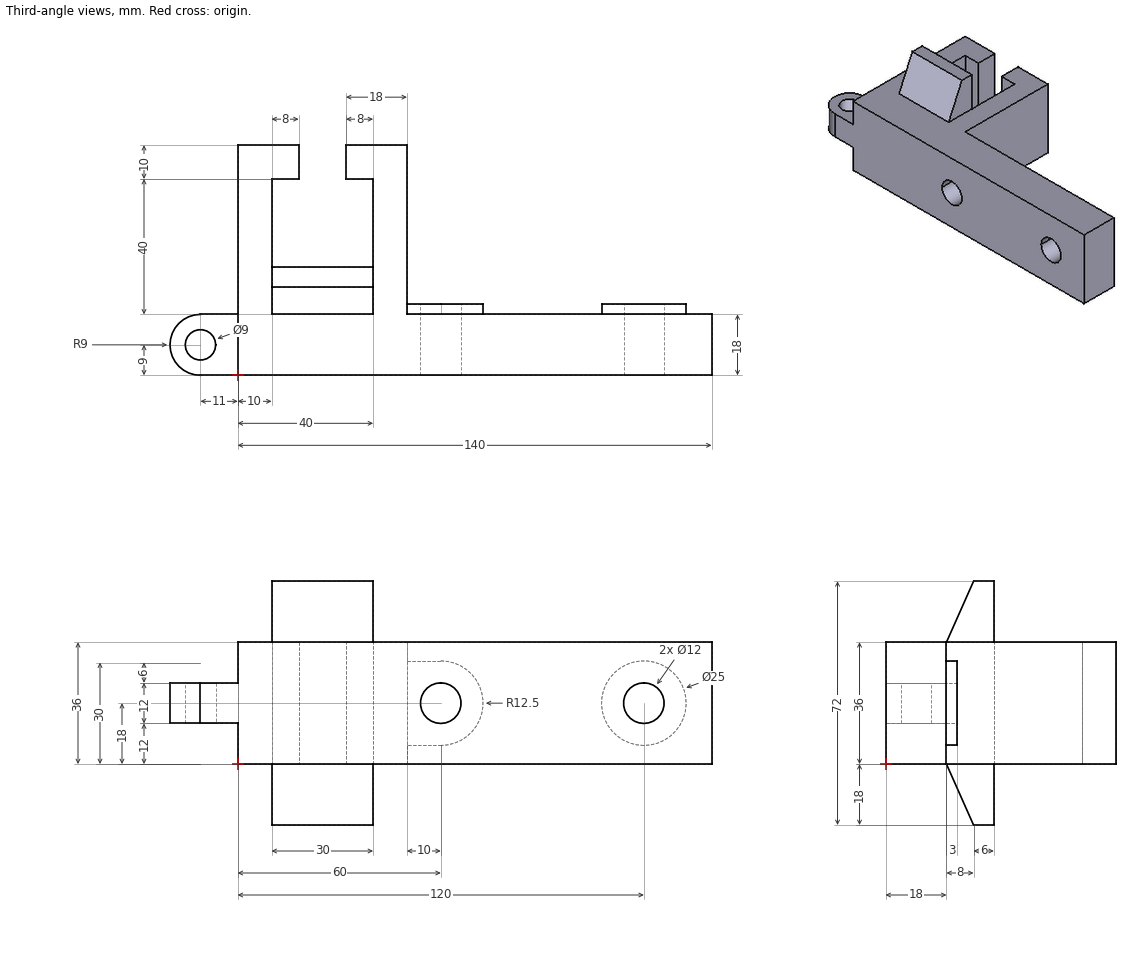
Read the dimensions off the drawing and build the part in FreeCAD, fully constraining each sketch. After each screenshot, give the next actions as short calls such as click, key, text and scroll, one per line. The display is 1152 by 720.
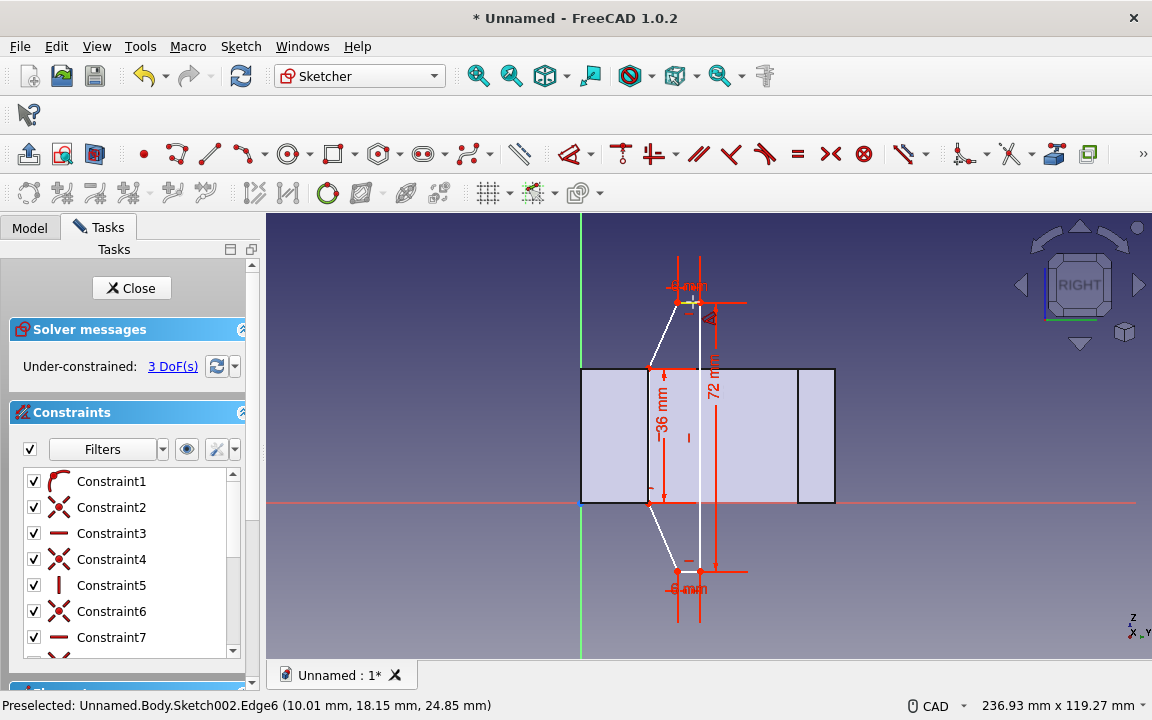
scroll(657, 524, up, 2)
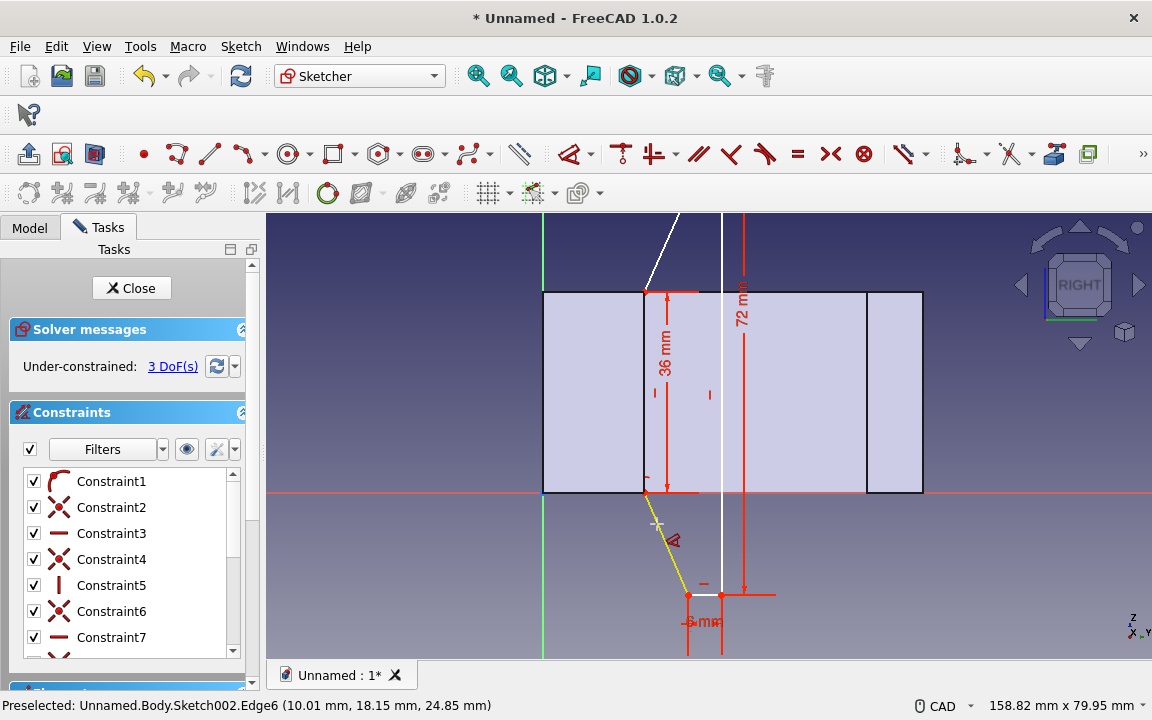
click(658, 524)
click(666, 459)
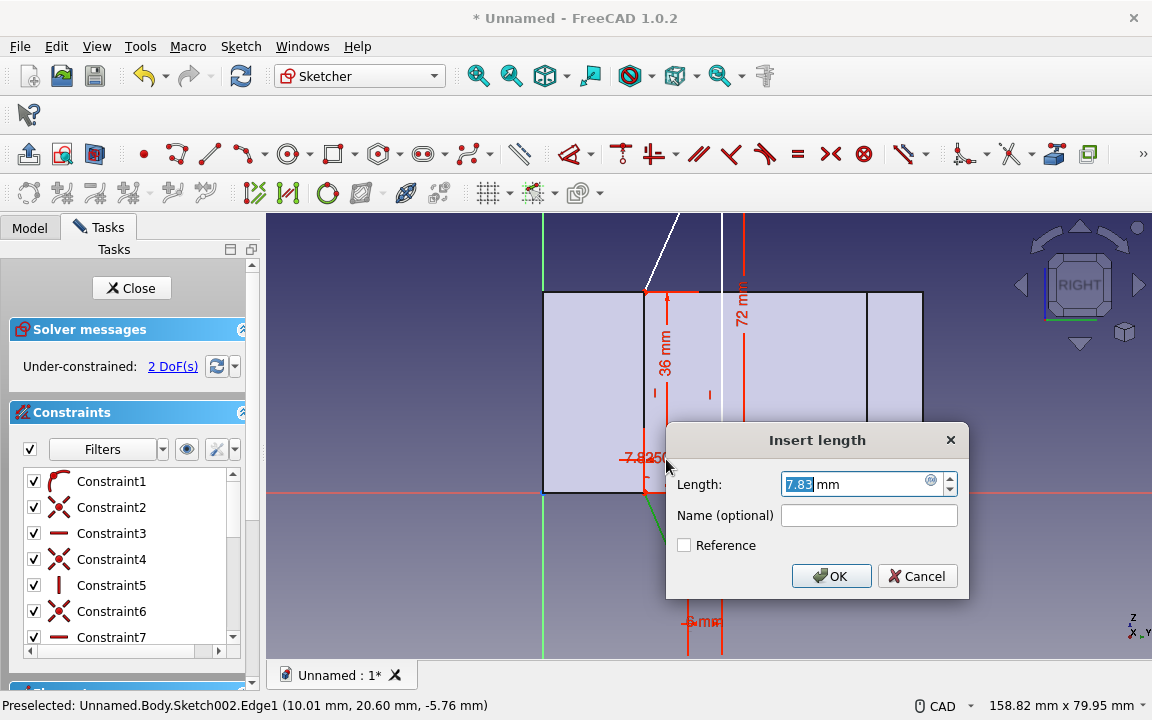
text(8)
key(Return)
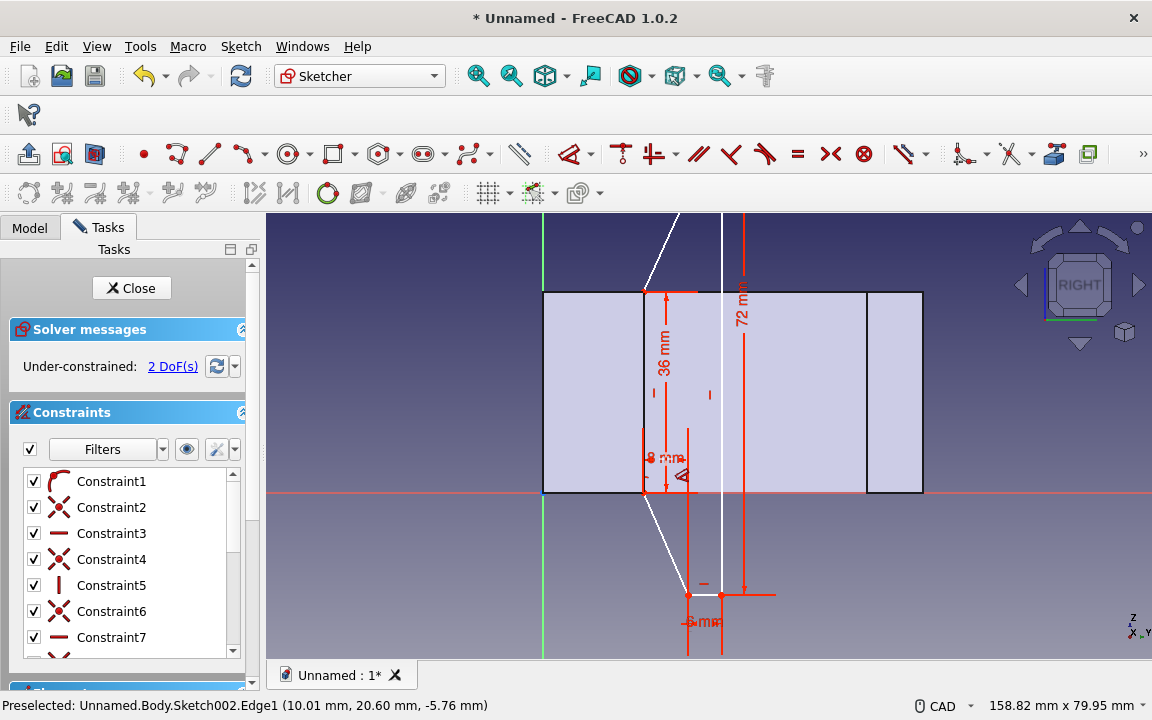
click(643, 493)
click(593, 527)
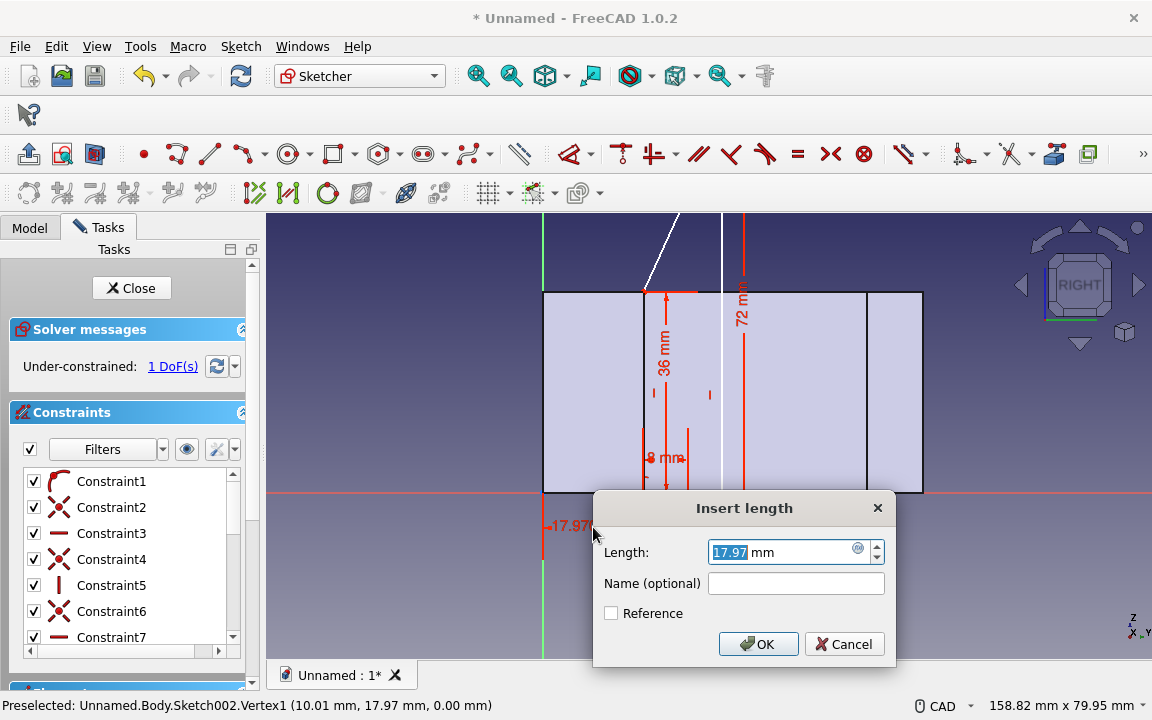
text(18)
key(Return)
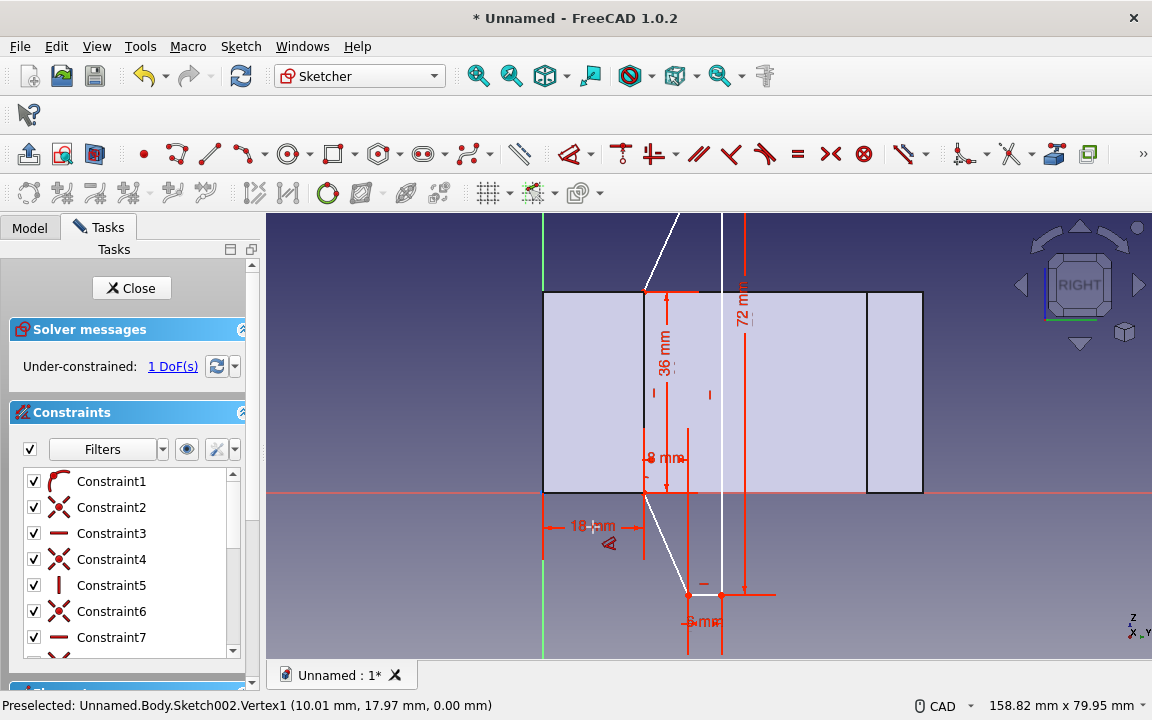
click(688, 595)
click(509, 544)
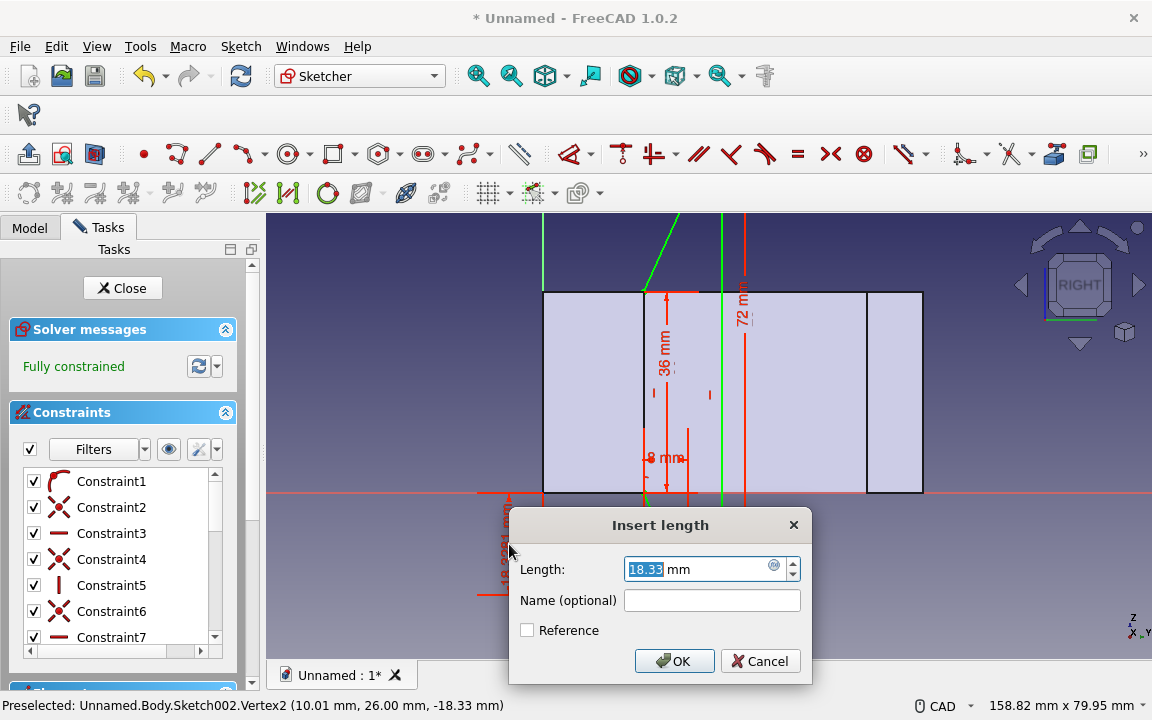
text(18)
key(Return)
key(Escape)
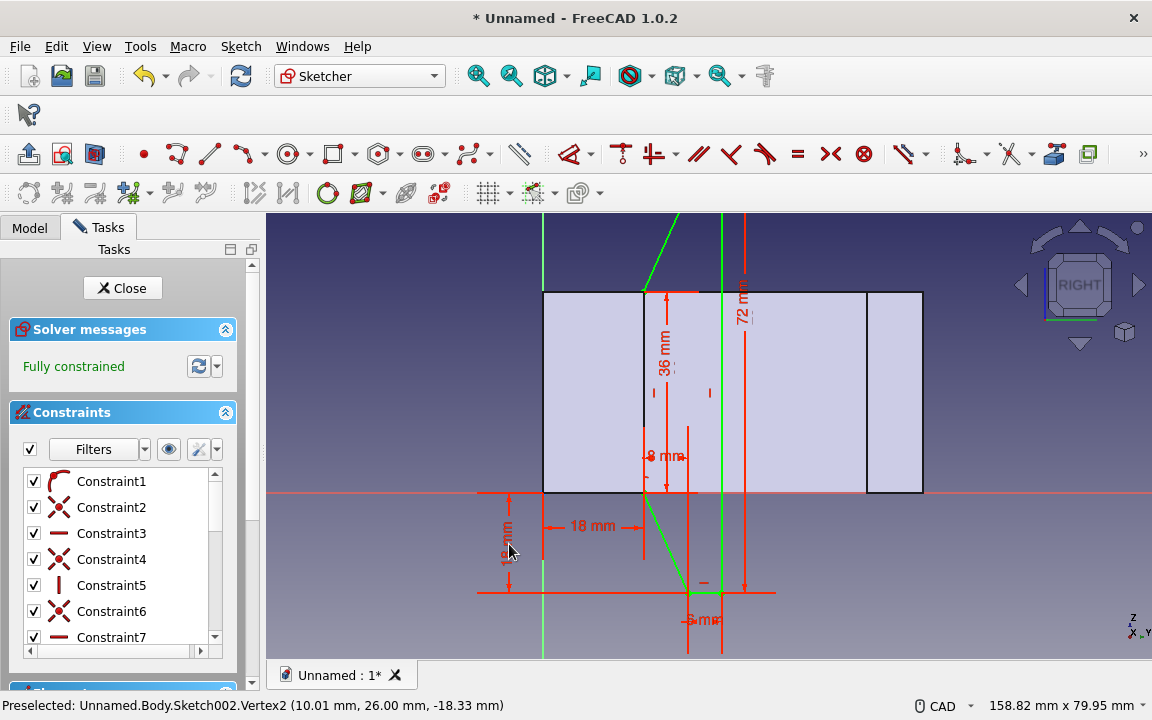
click(123, 288)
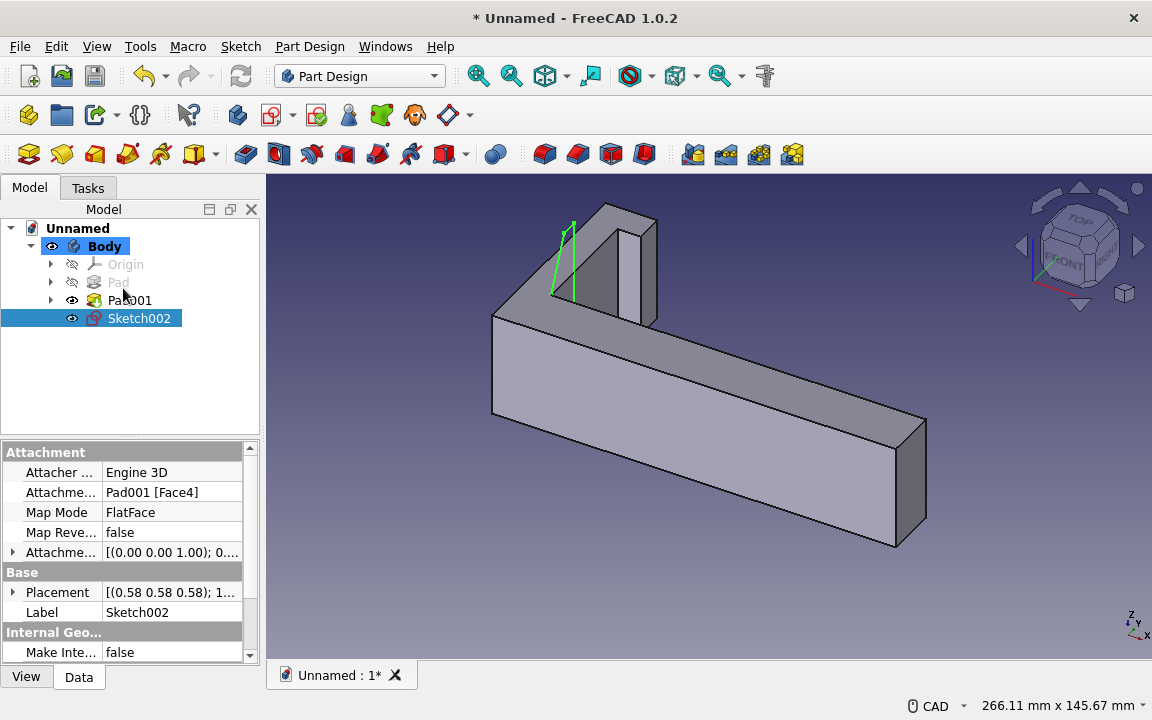
click(29, 154)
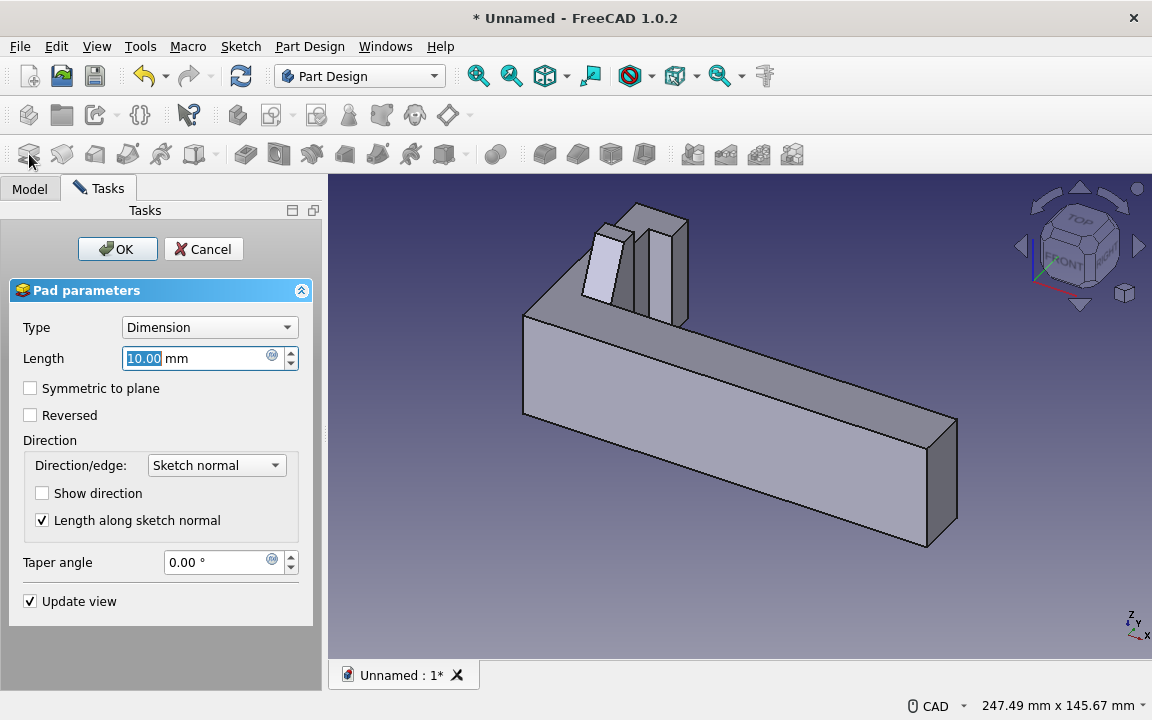
text(30)
key(Tab)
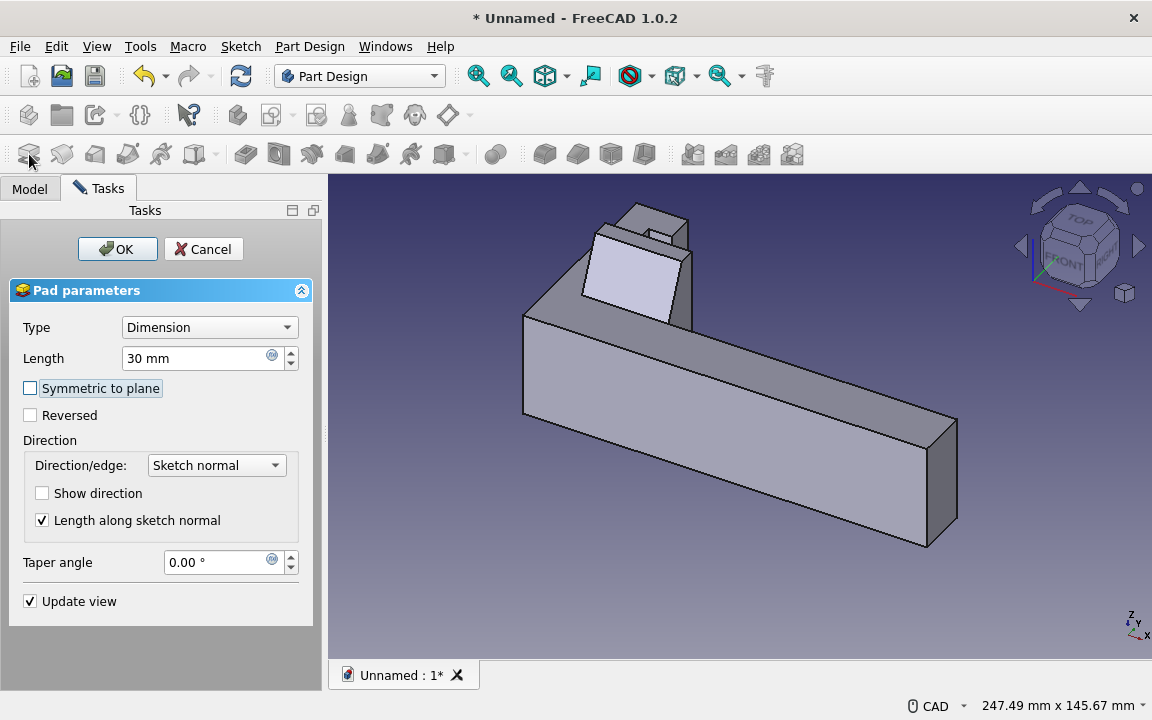
click(118, 249)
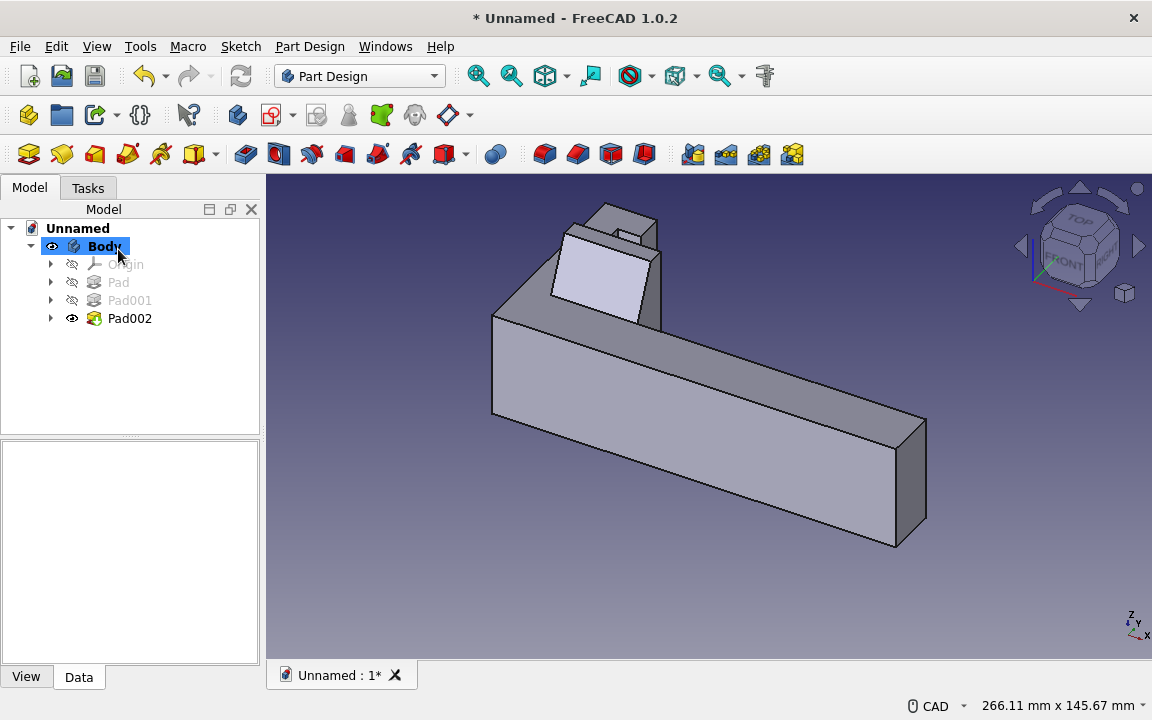
key(v)
key(f)